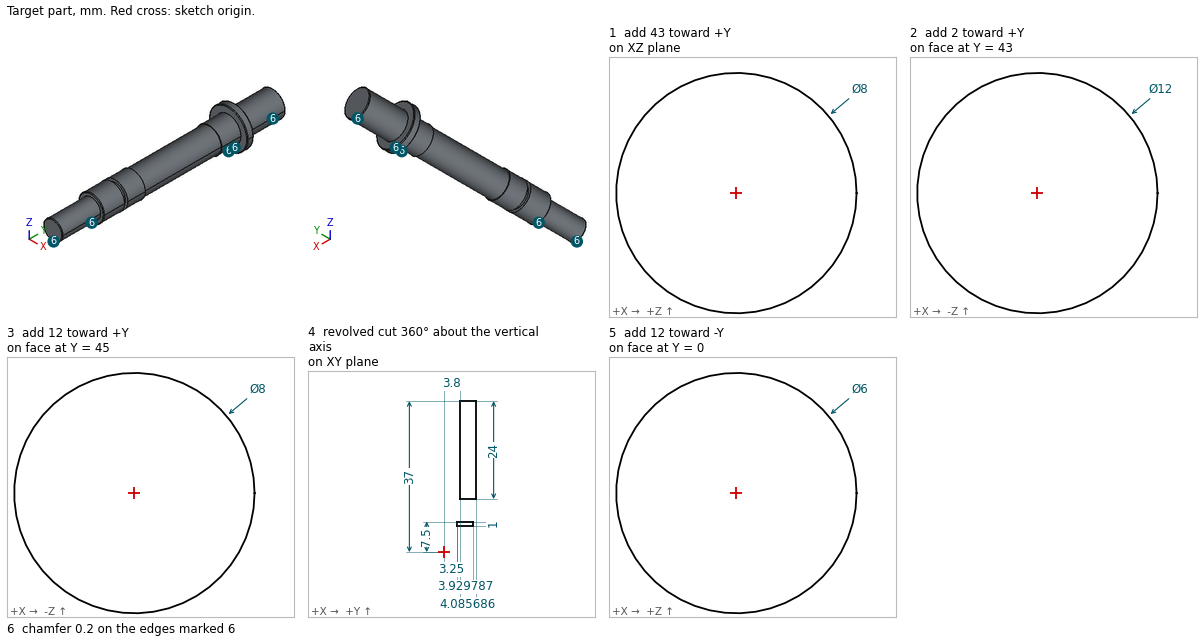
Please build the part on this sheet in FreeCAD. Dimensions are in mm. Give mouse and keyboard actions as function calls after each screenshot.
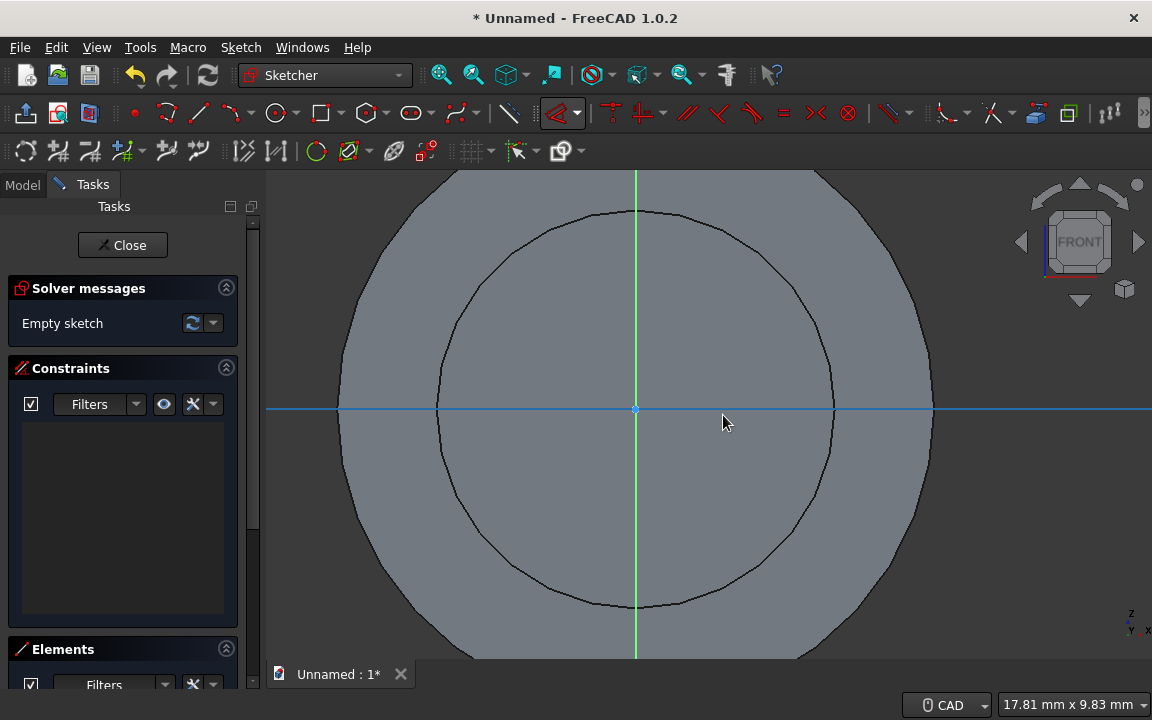
click(276, 114)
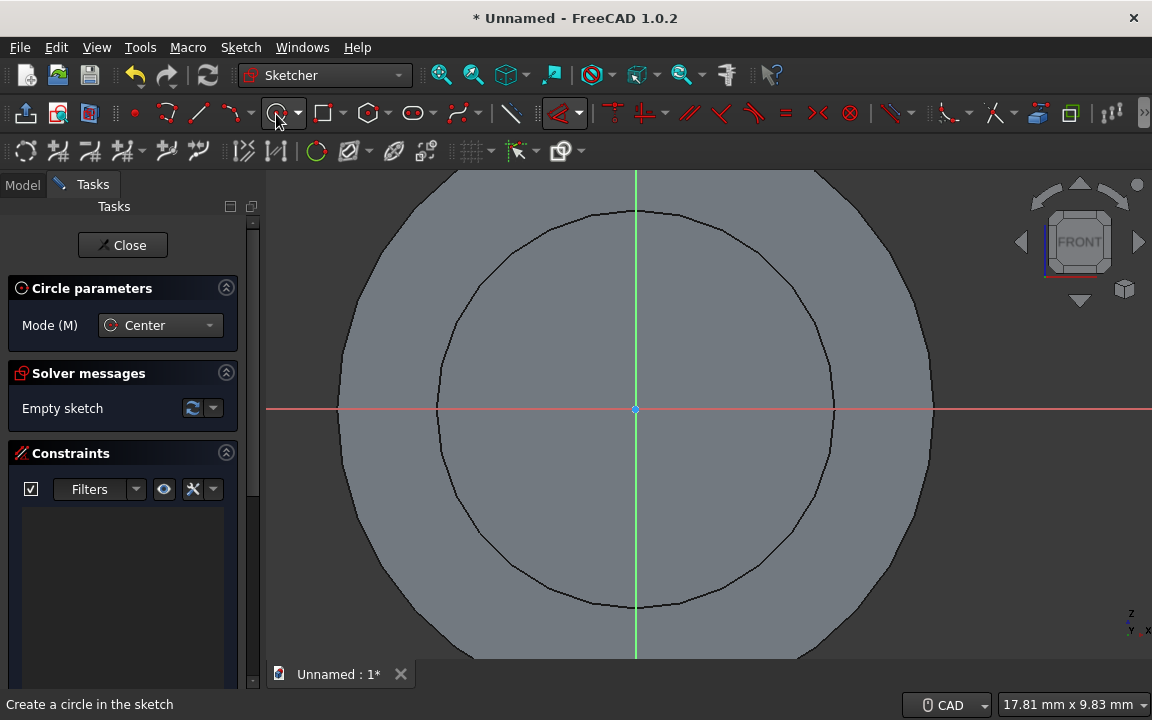
click(636, 409)
move(741, 304)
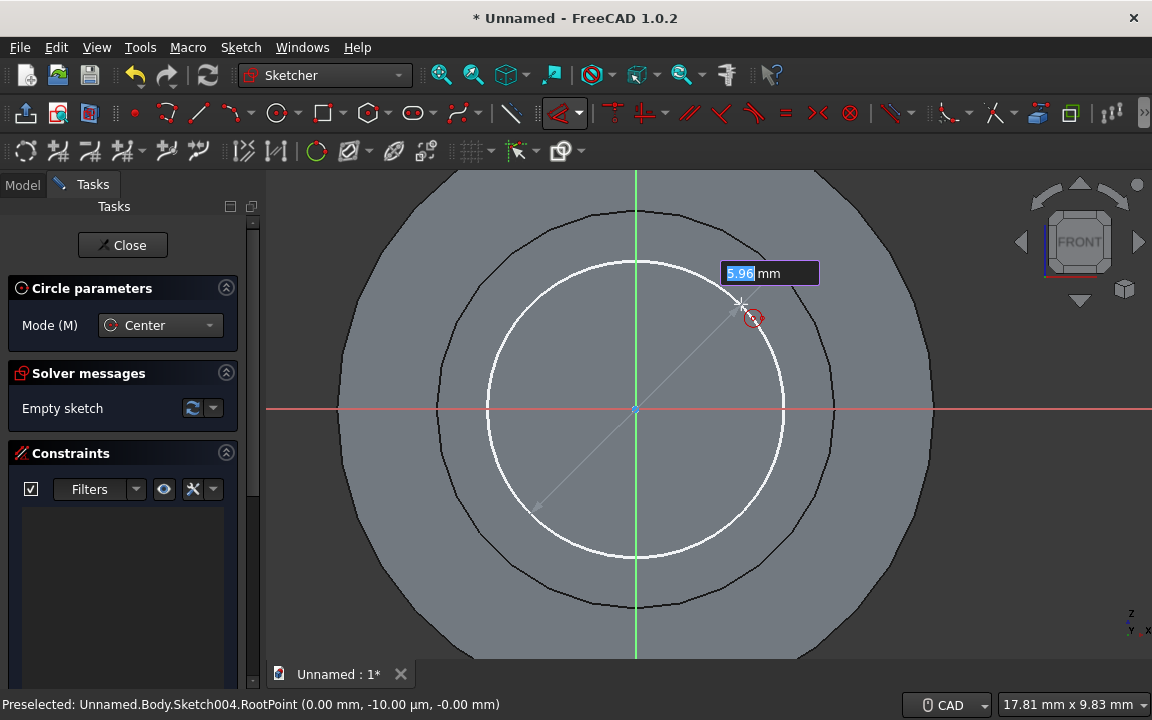
text(6)
key(Return)
key(Escape)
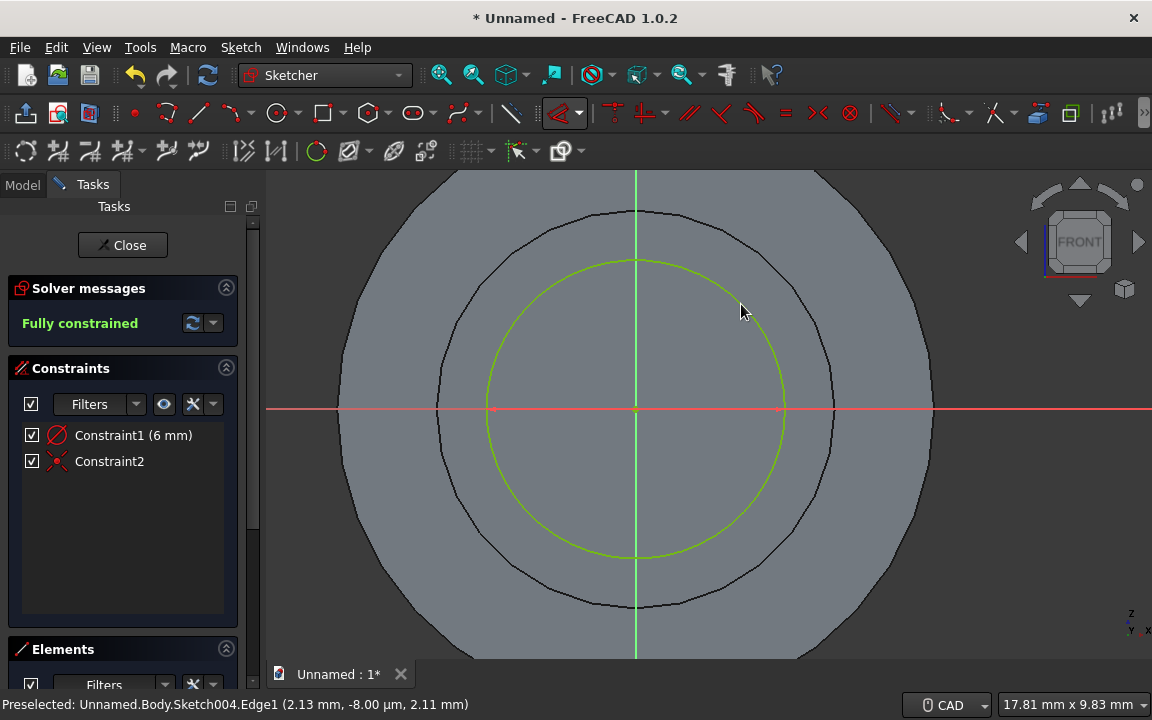
click(123, 245)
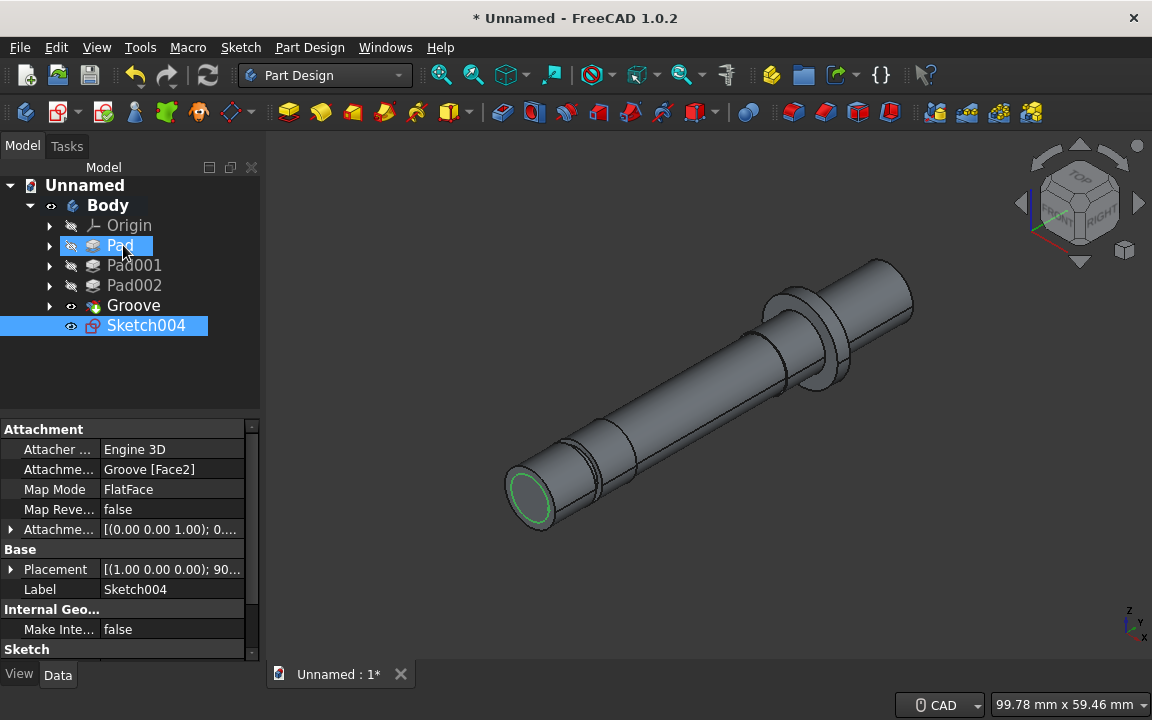
click(290, 112)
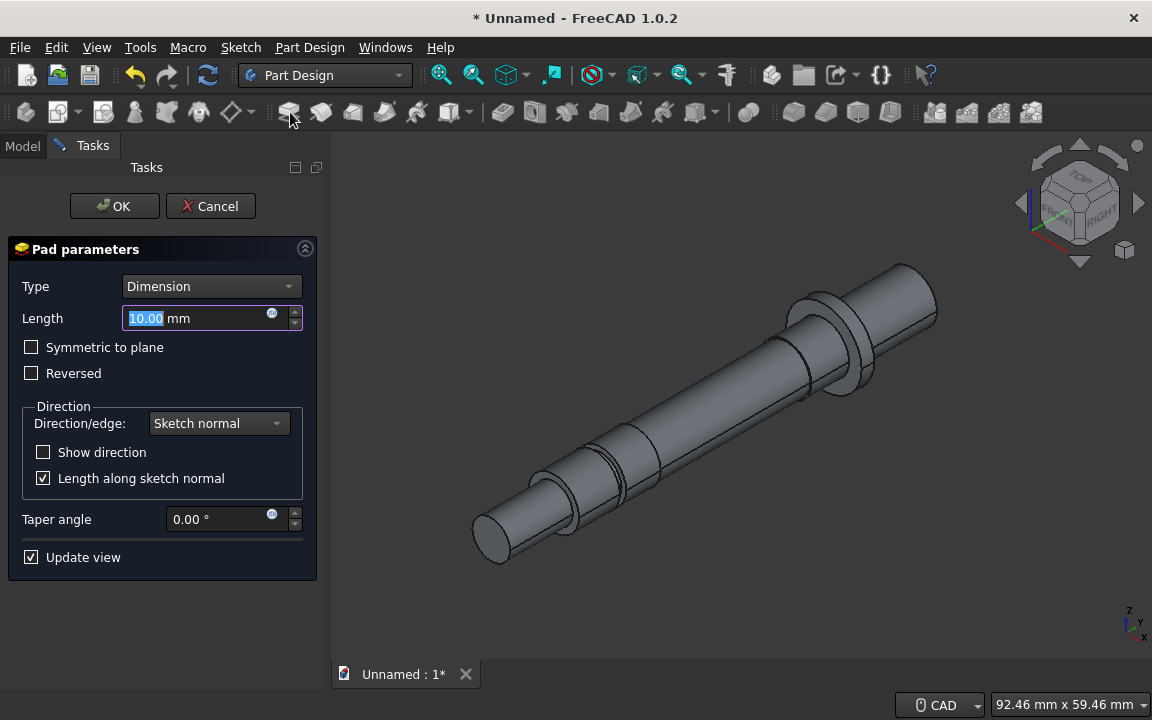
text(12)
key(Tab)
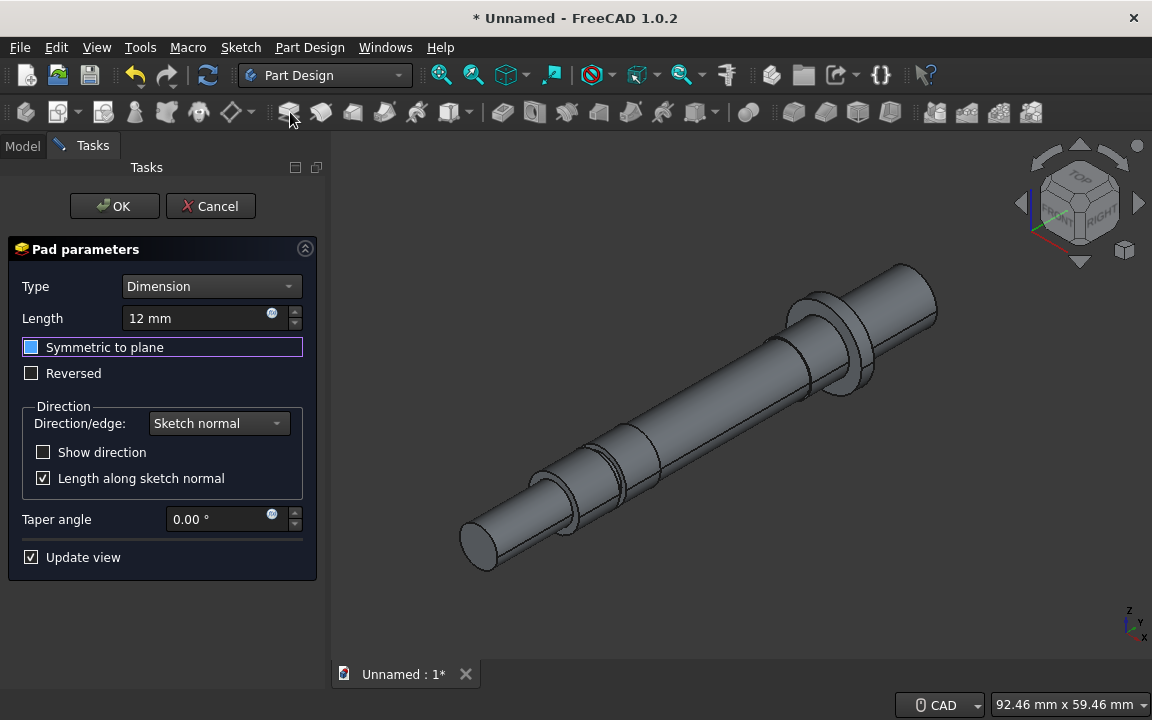
click(115, 206)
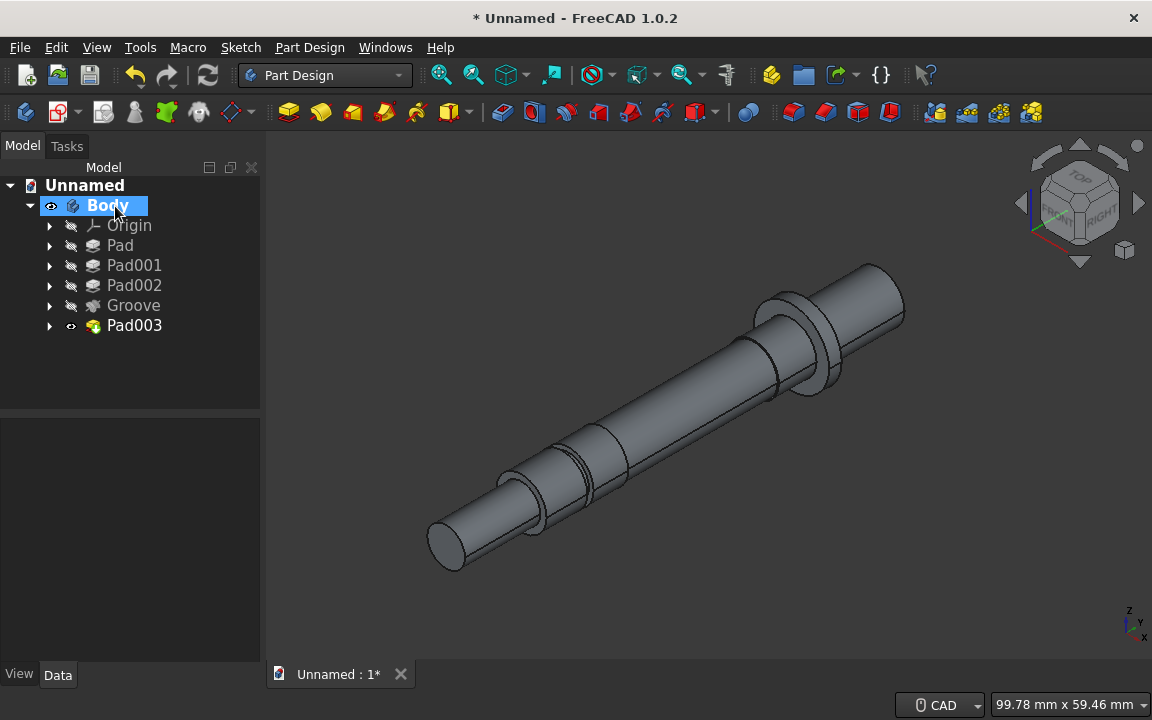
click(501, 473)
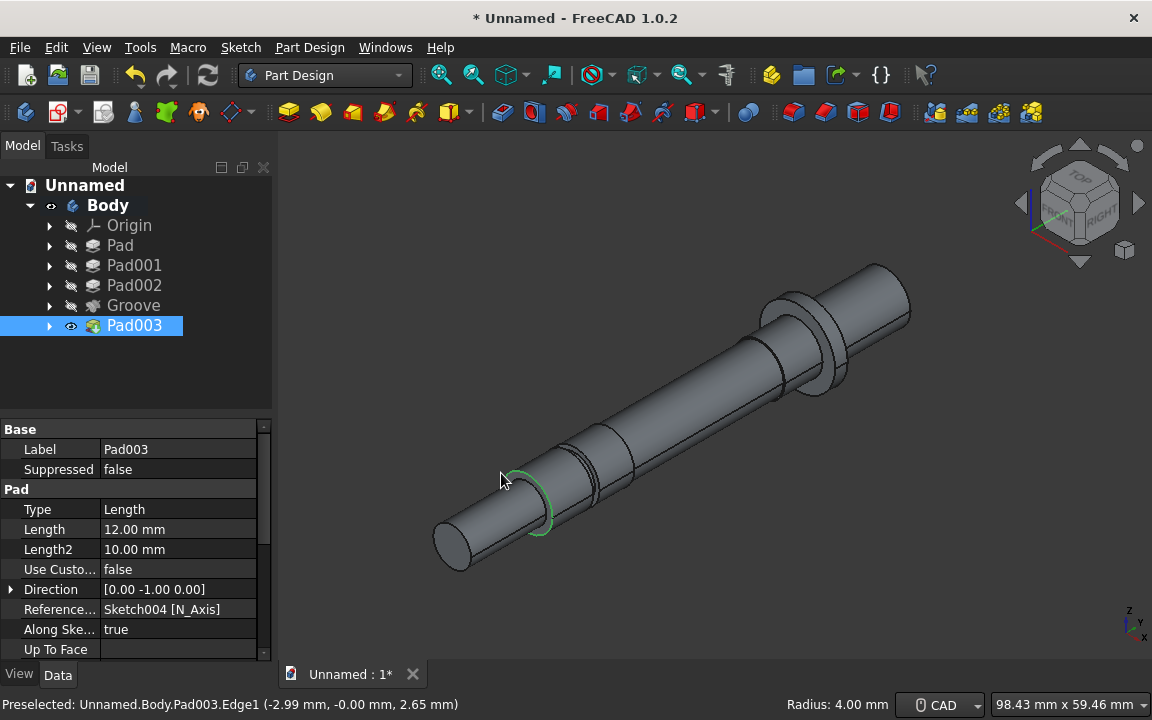
click(437, 524, ctrl)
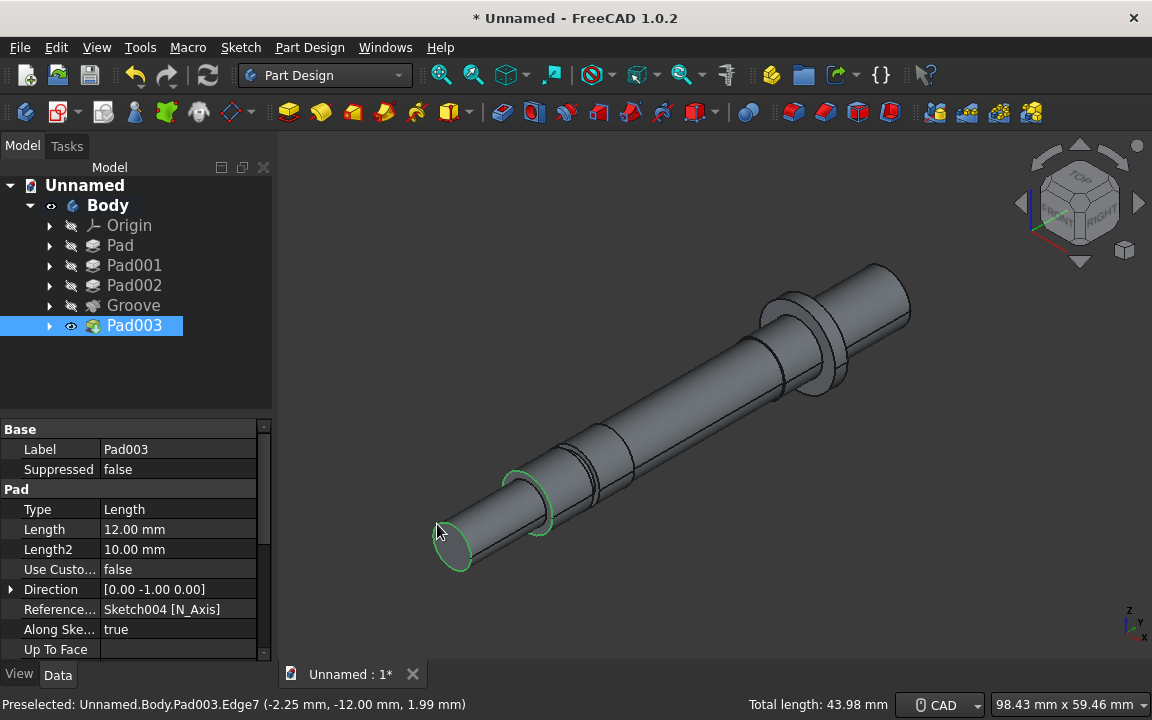
click(786, 298, ctrl)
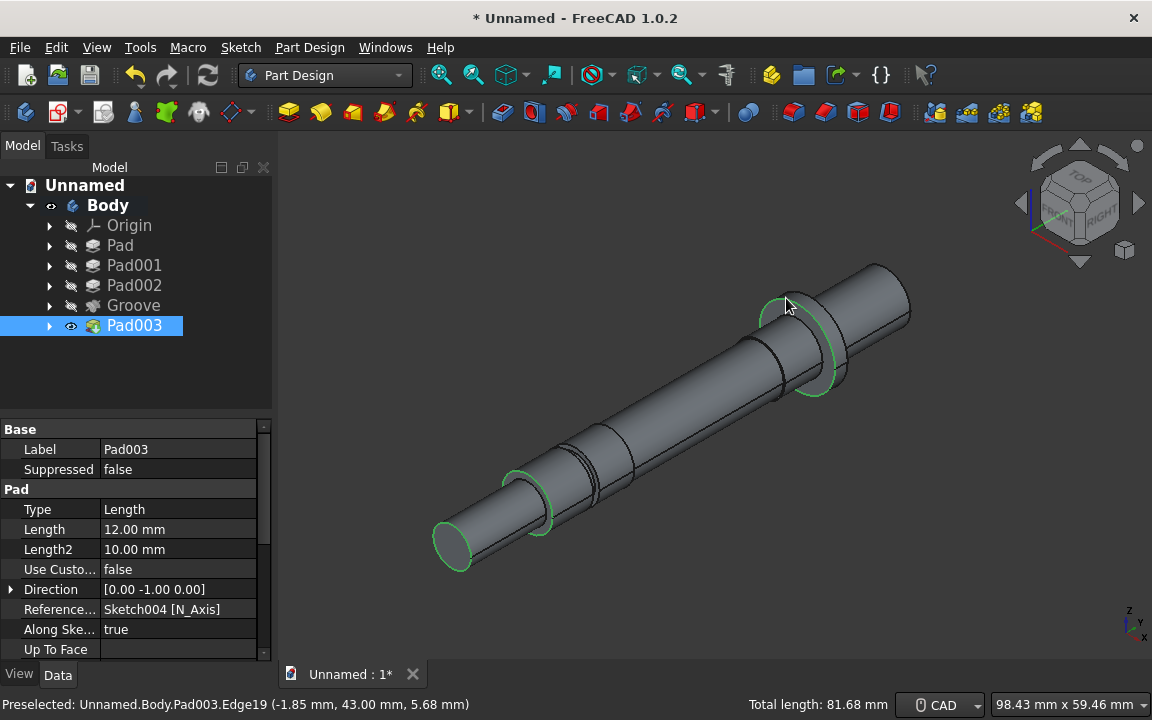
click(822, 304, ctrl)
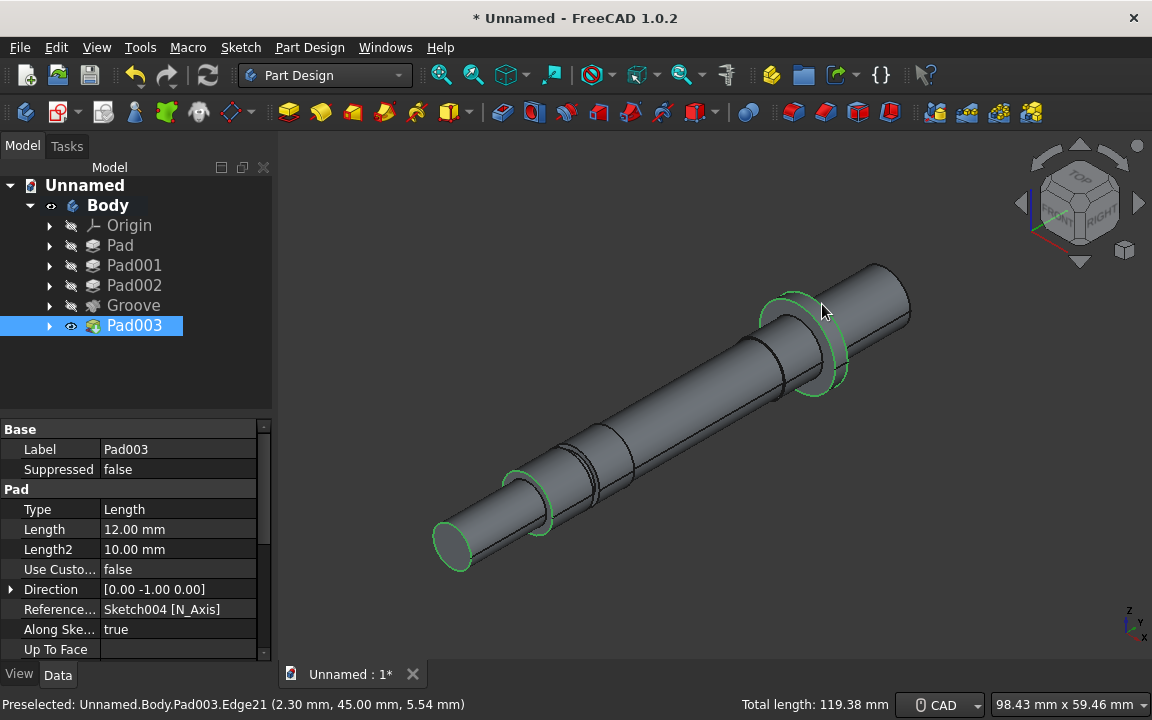
key(2)